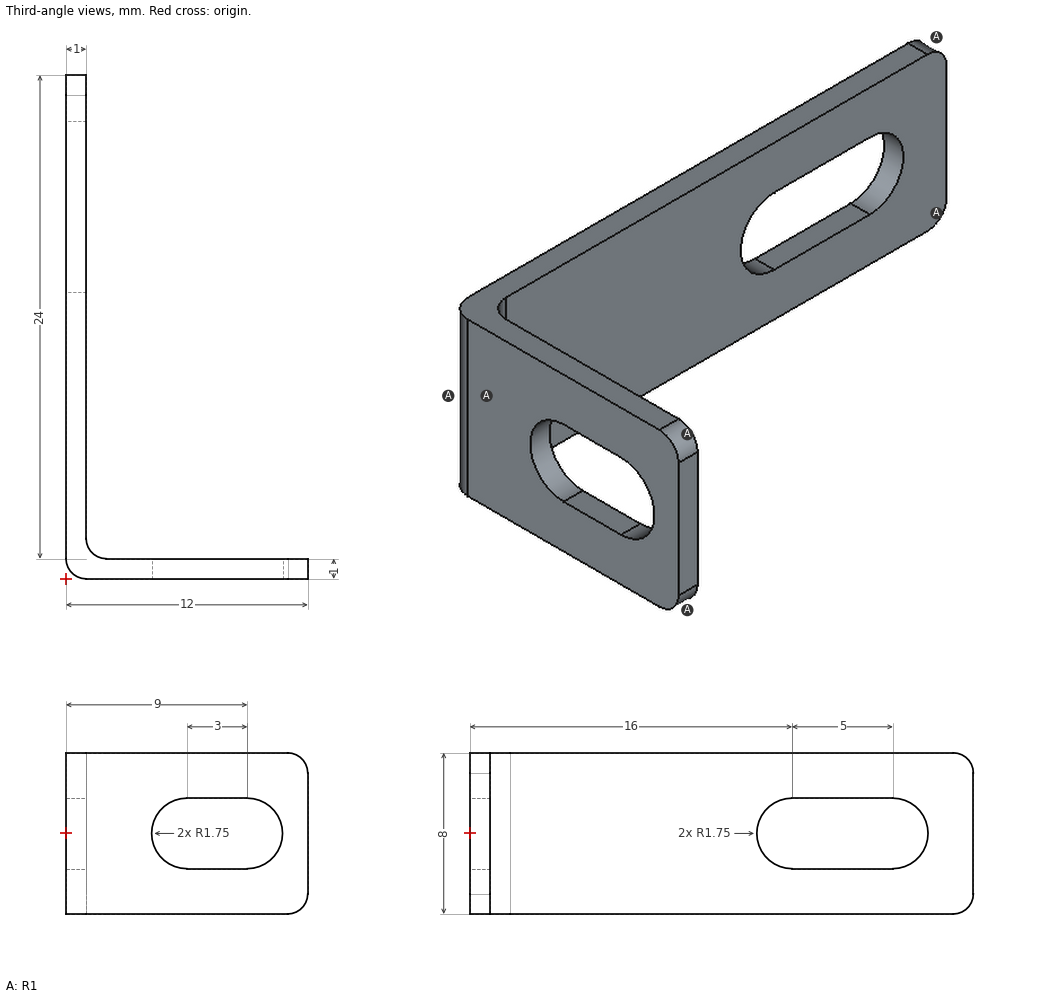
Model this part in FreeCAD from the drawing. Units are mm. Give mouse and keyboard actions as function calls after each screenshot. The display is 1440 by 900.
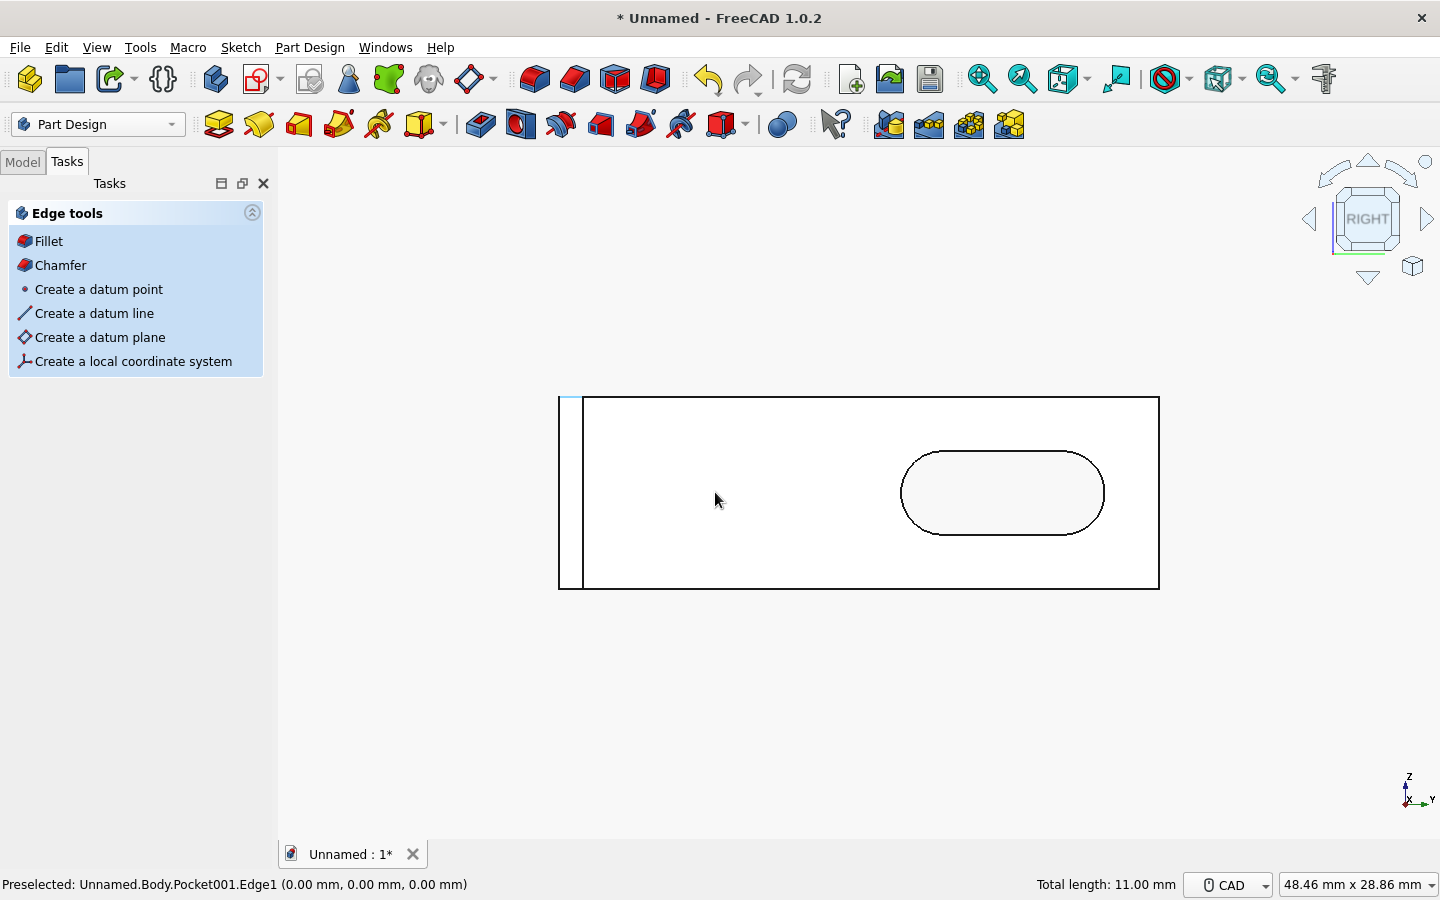
click(571, 588, ctrl)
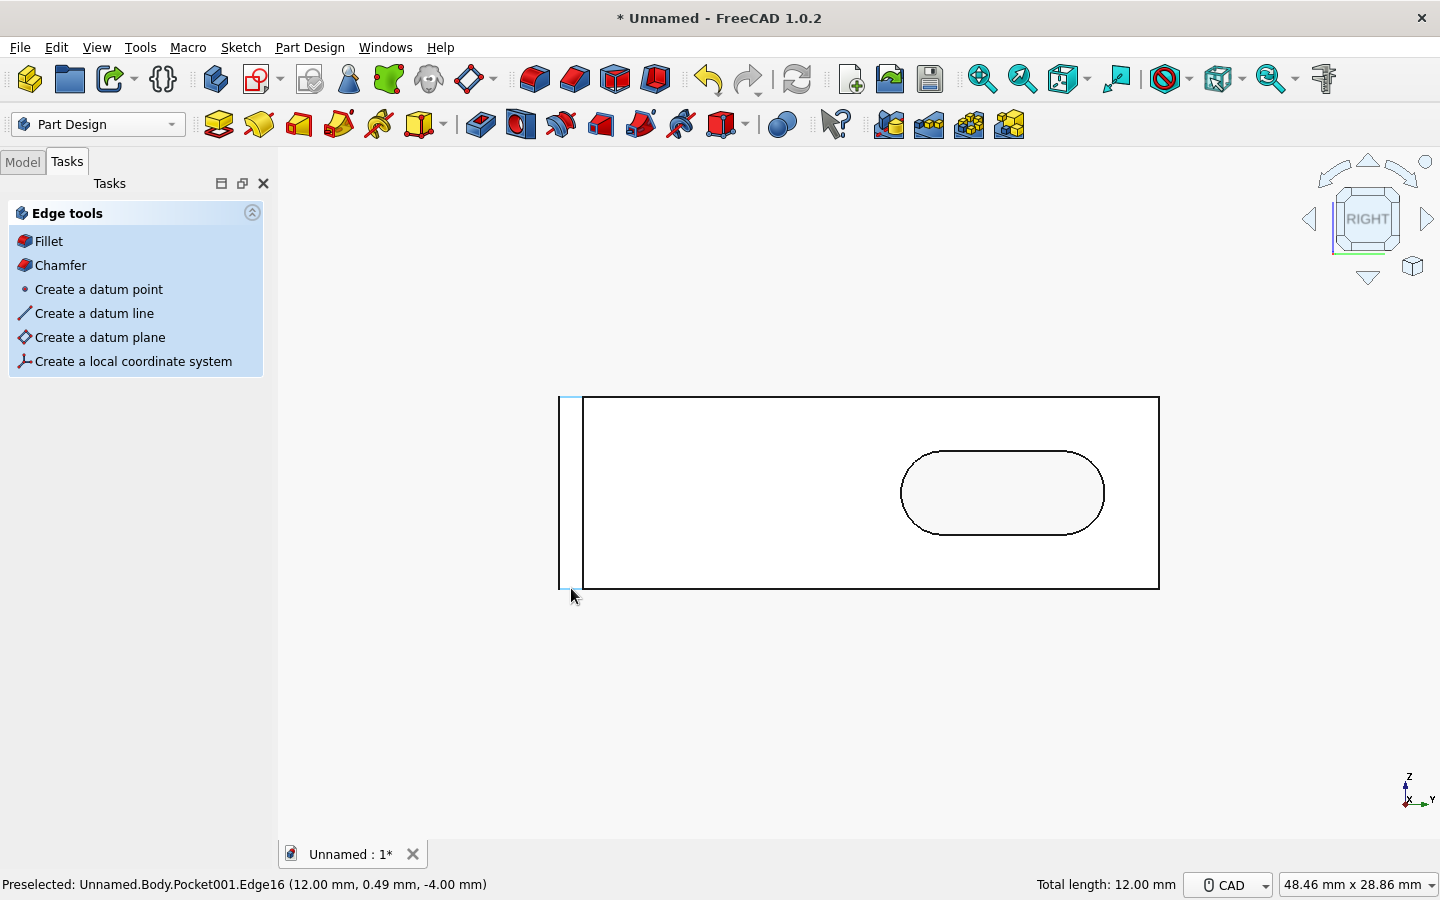
key(5)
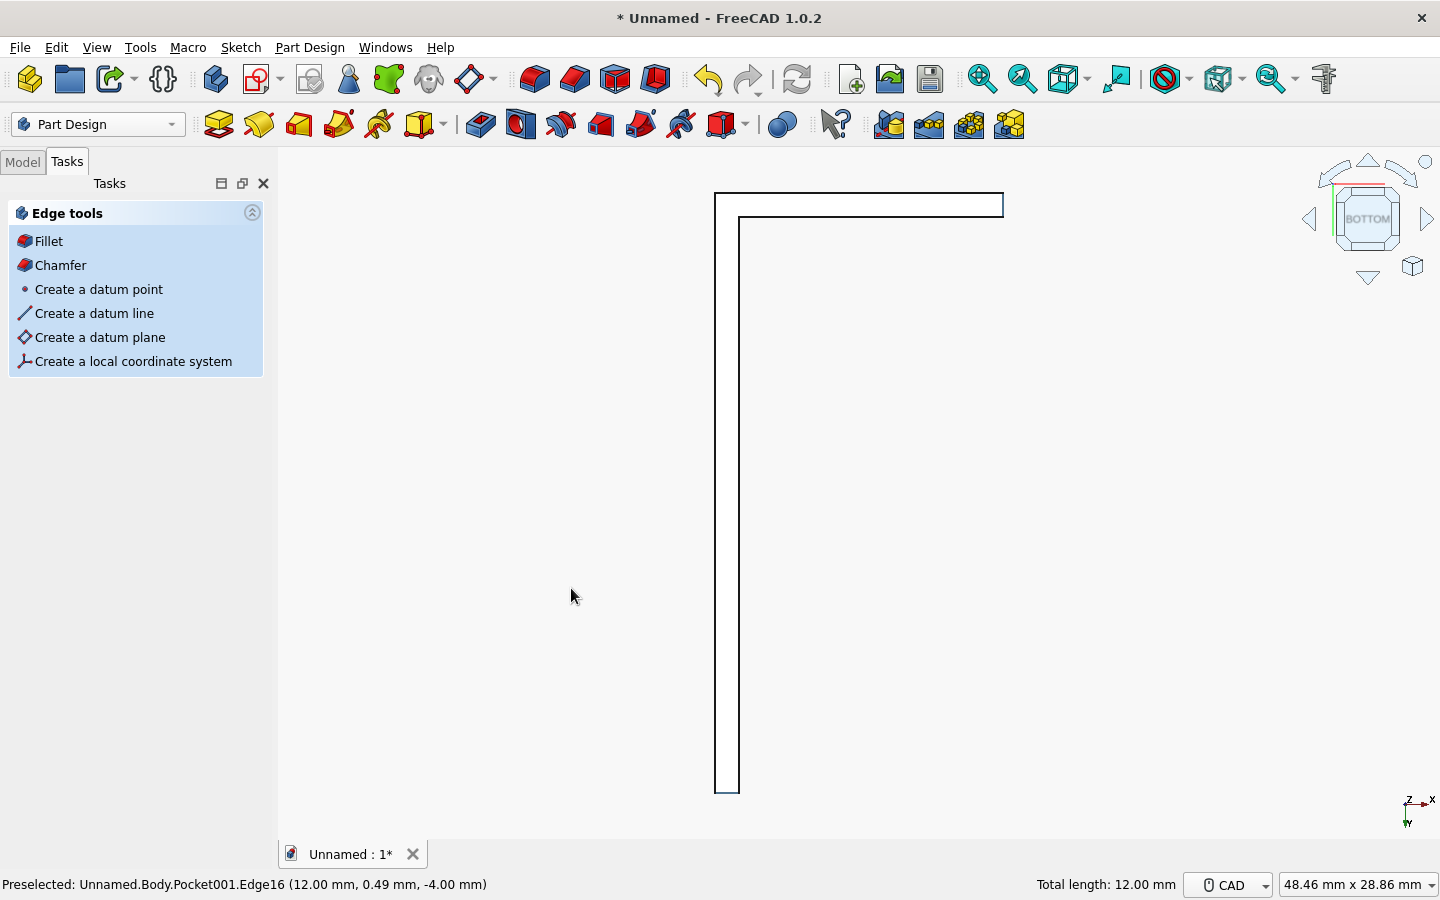
key(4)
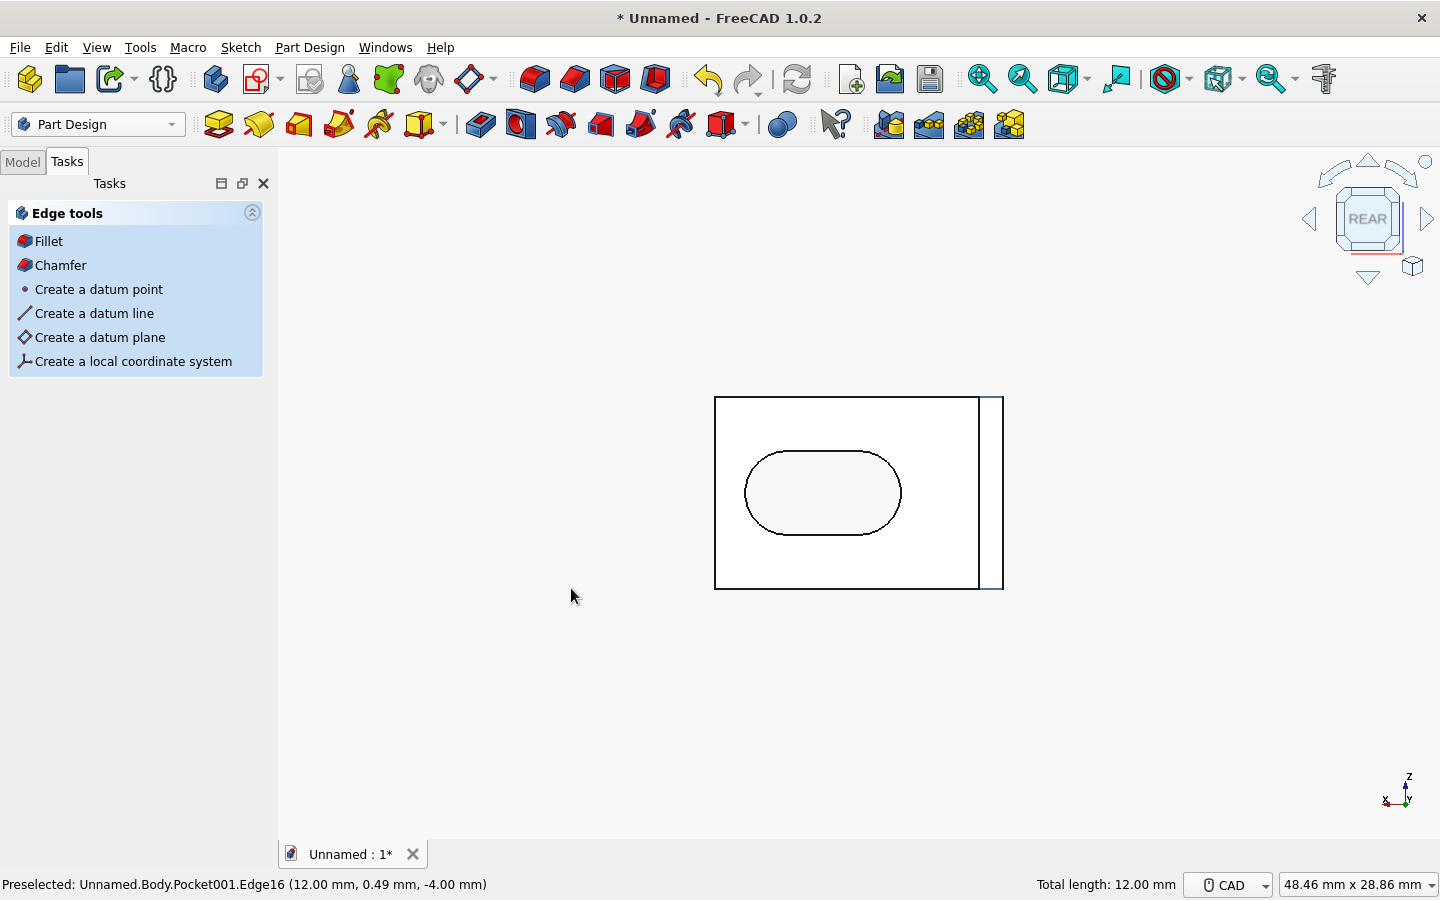
key(v)
key(f)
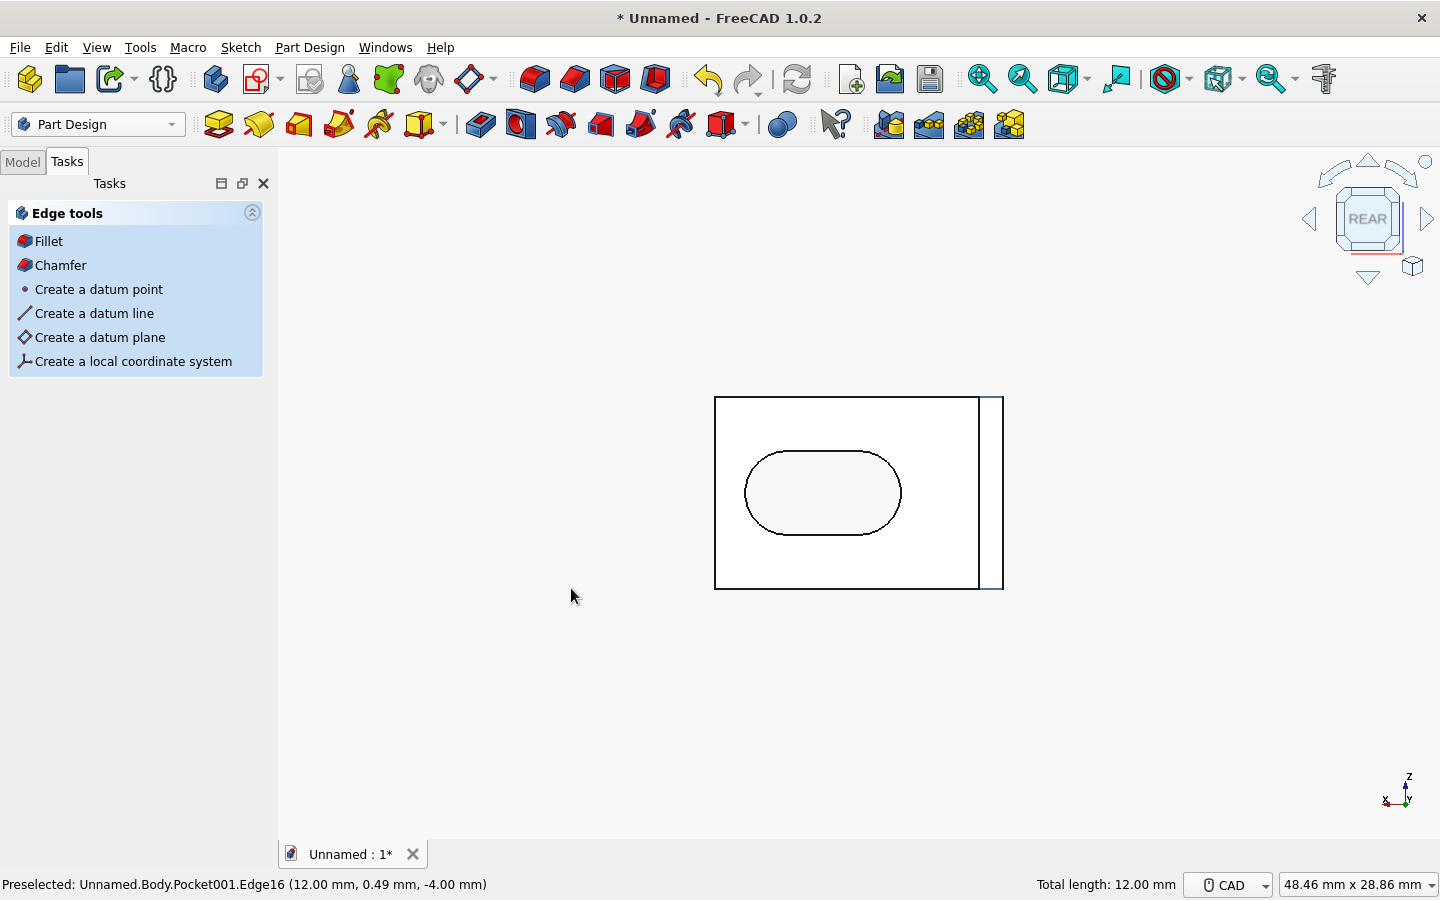
key(6)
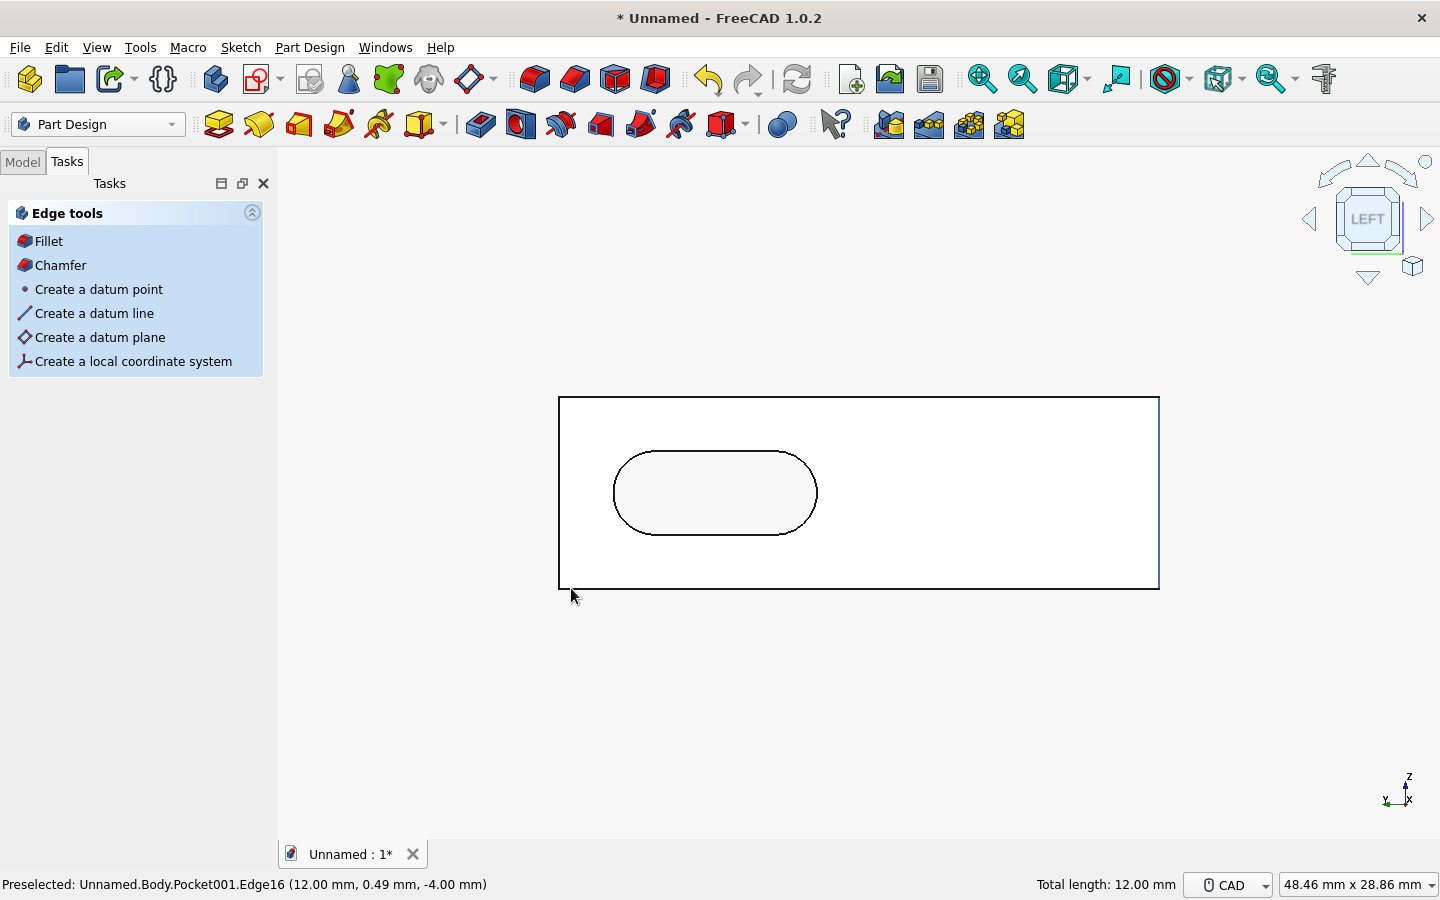
key(v)
key(3)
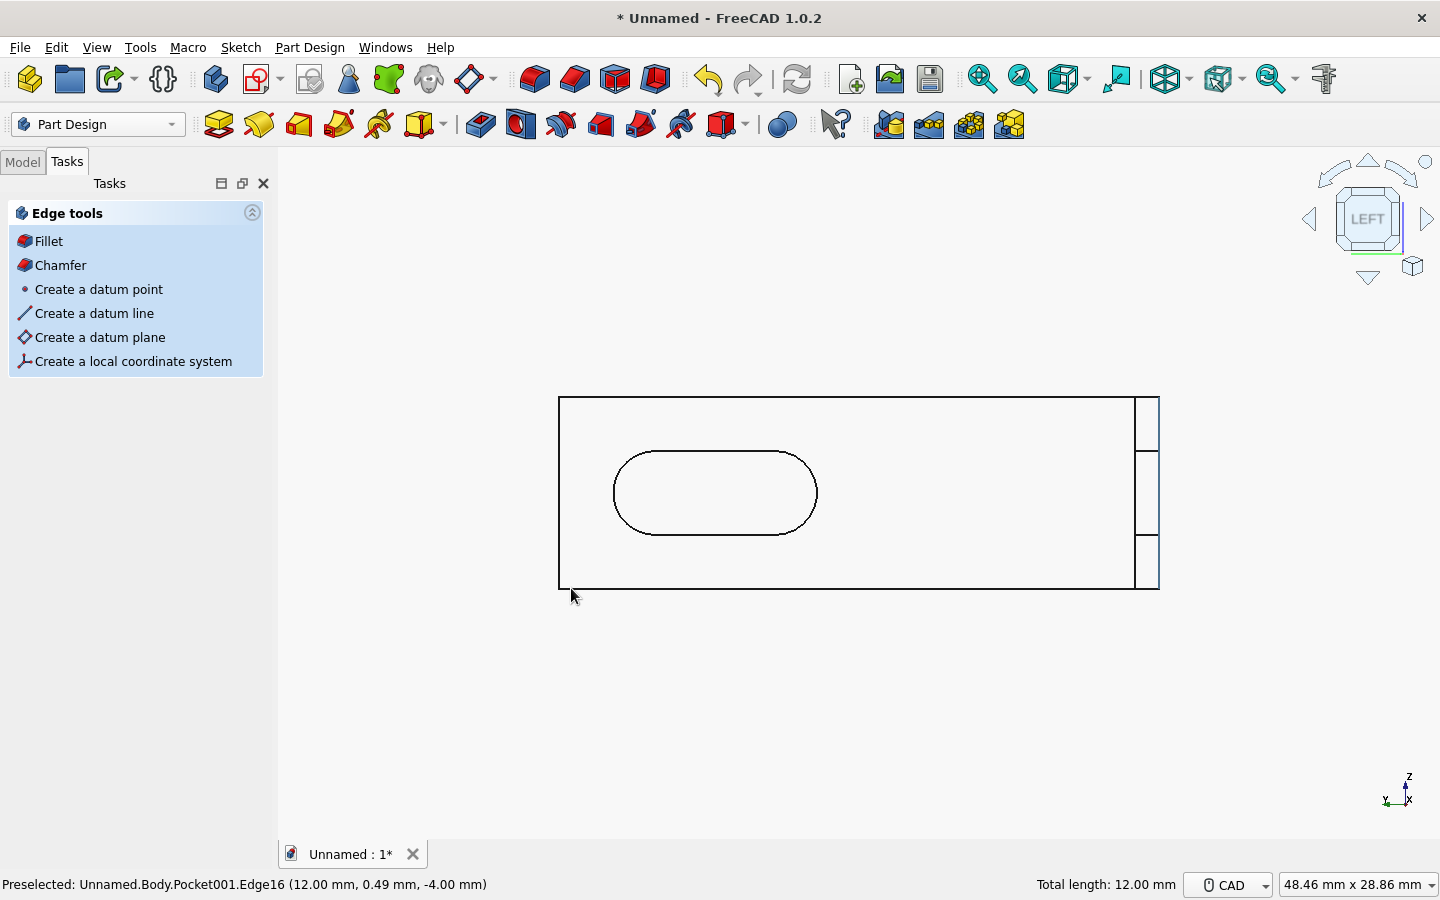
key(0)